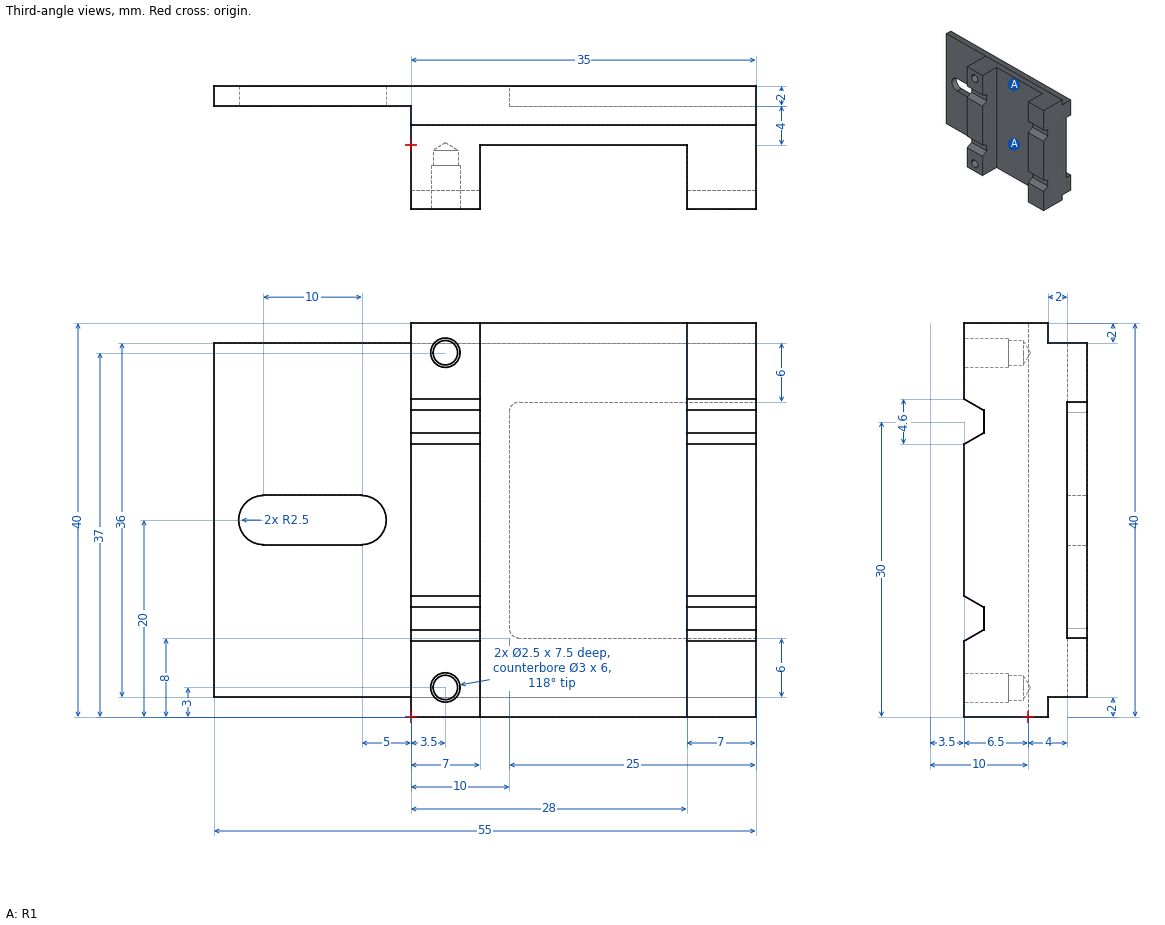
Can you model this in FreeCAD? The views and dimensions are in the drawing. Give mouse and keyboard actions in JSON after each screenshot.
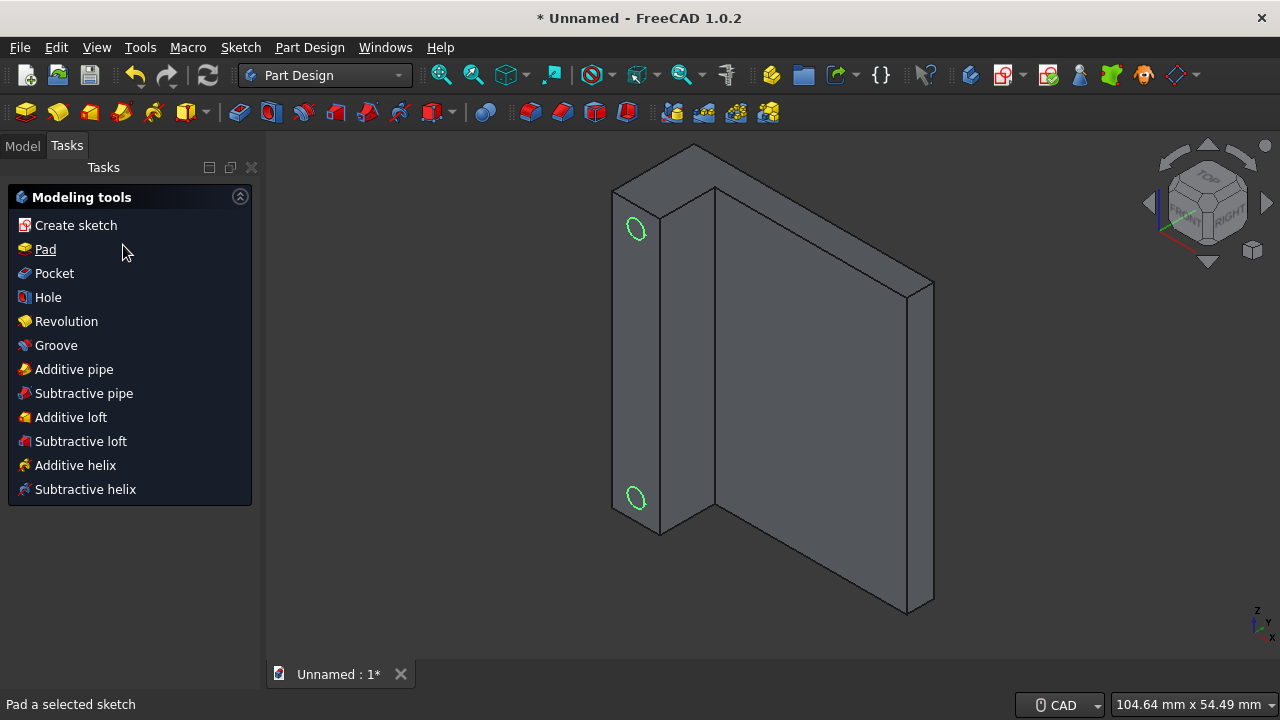
{"action": "left_click", "coordinate": [272, 112]}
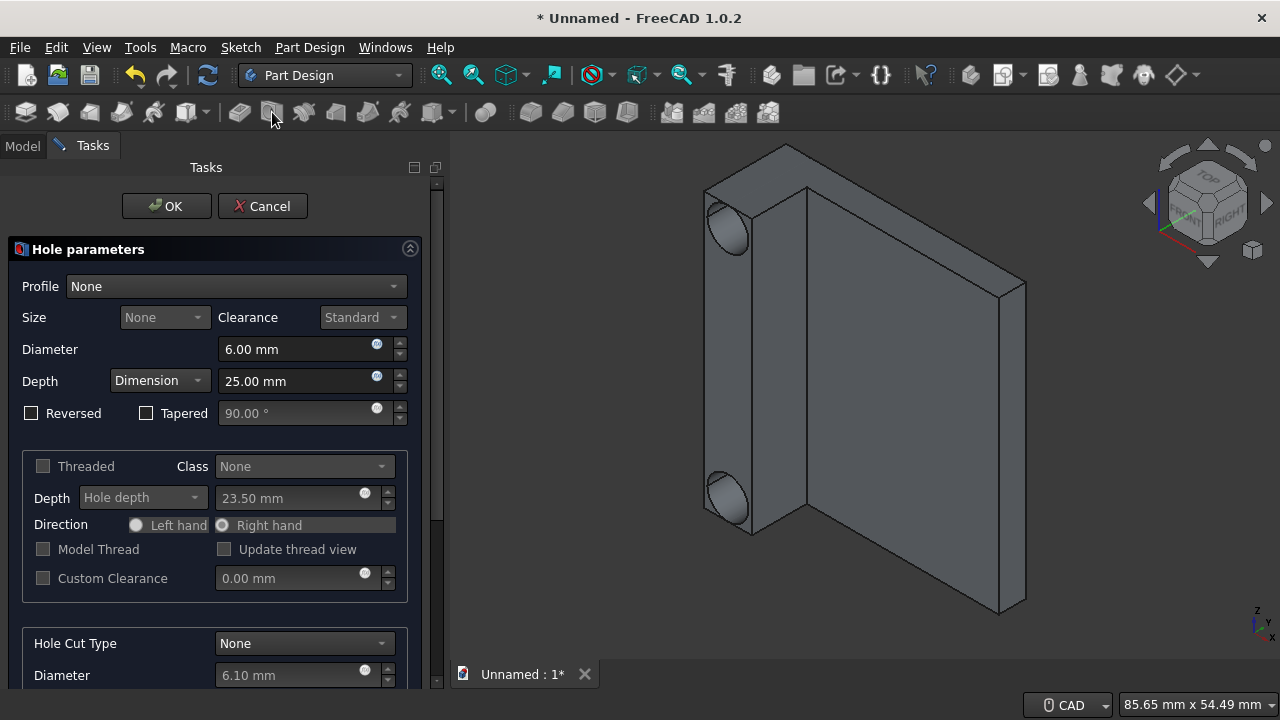
{"action": "triple_click", "coordinate": [305, 349]}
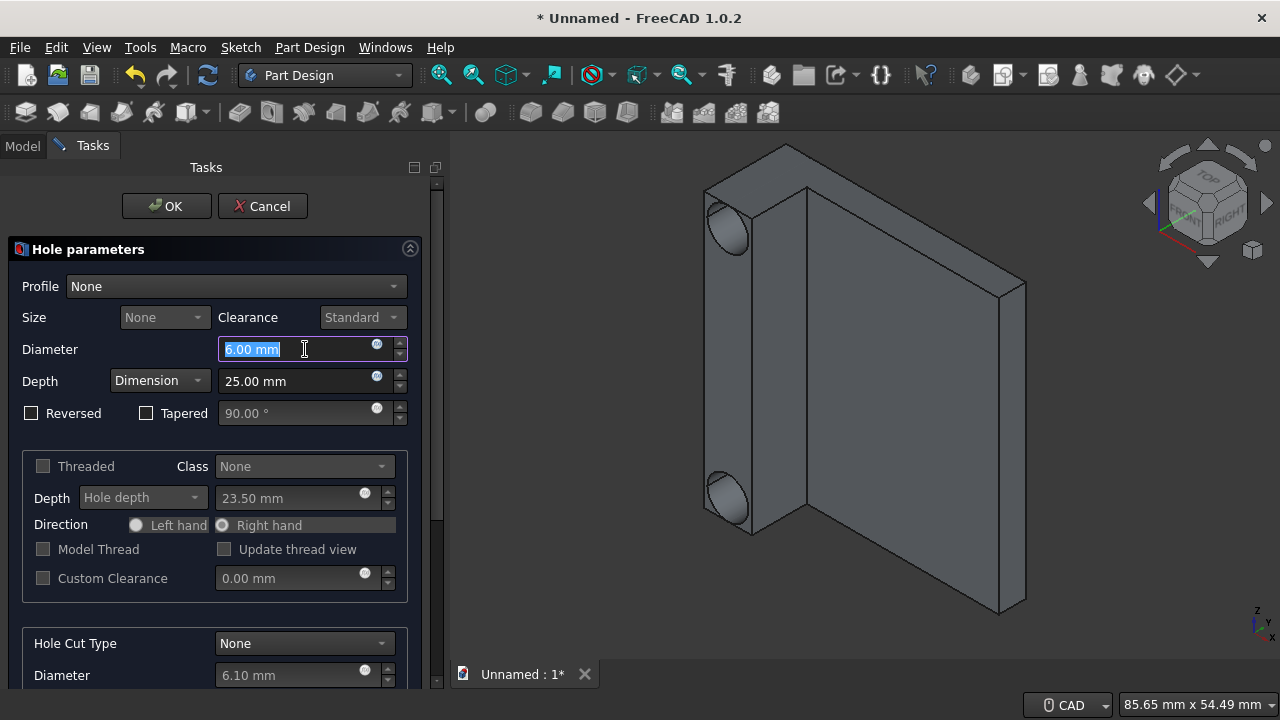
{"action": "type", "text": "2.5"}
{"action": "key", "text": "Tab"}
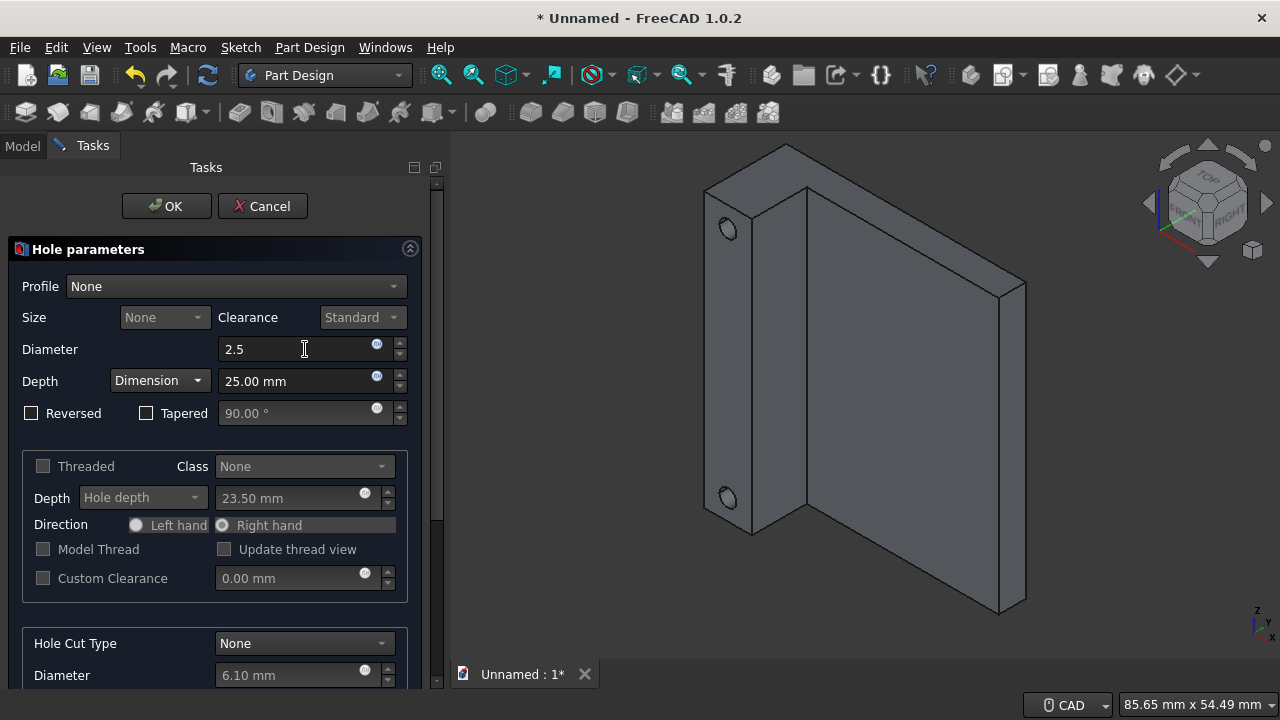
{"action": "triple_click", "coordinate": [305, 381]}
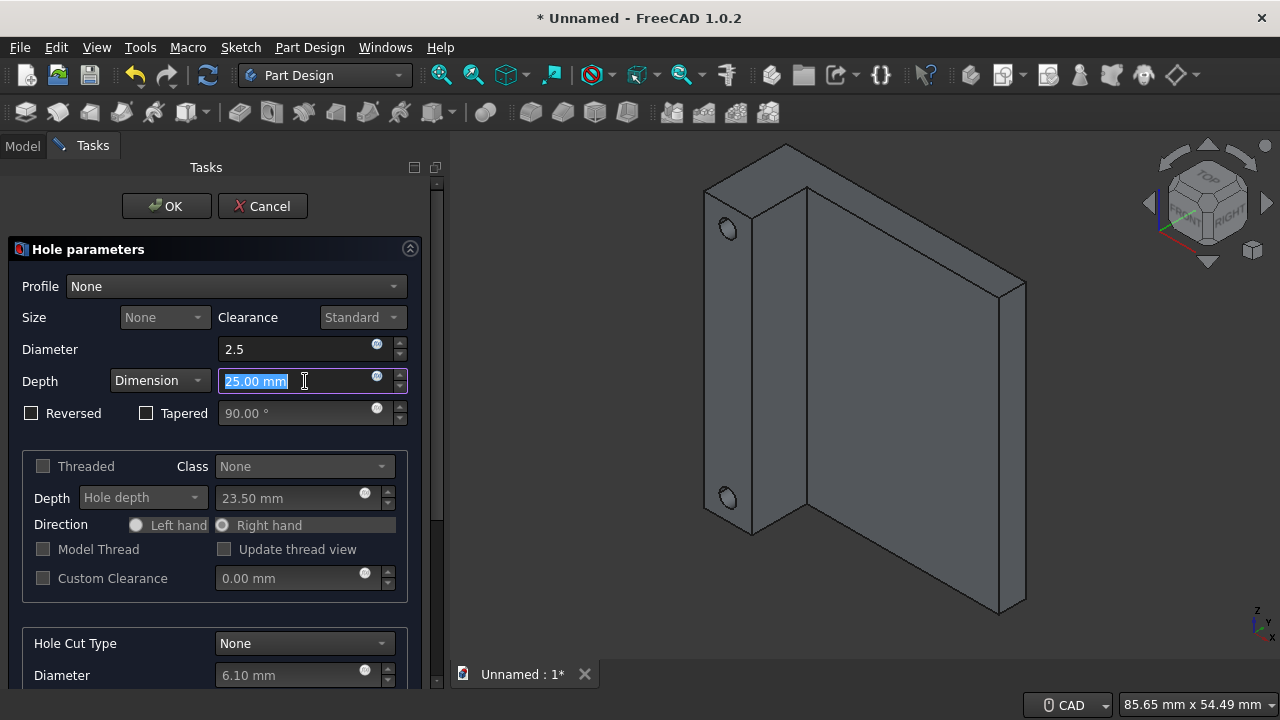
{"action": "type", "text": "7.5"}
{"action": "key", "text": "Tab"}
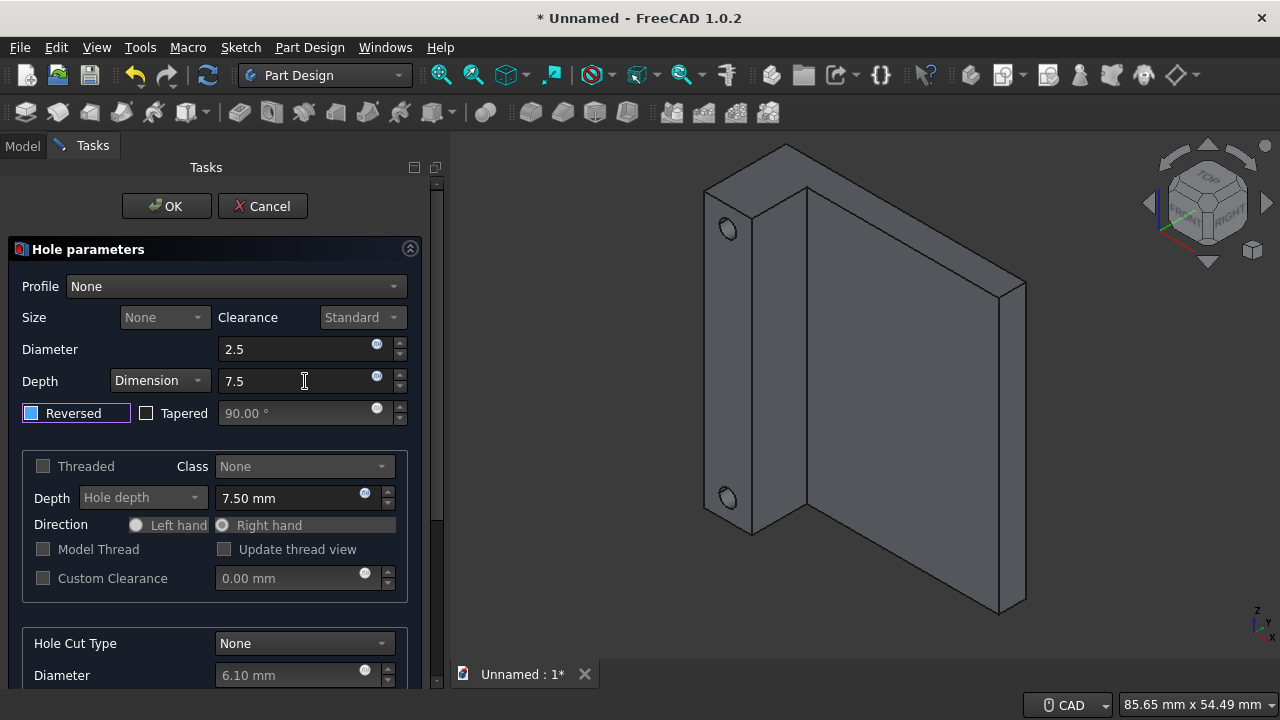
{"action": "left_click", "coordinate": [306, 644]}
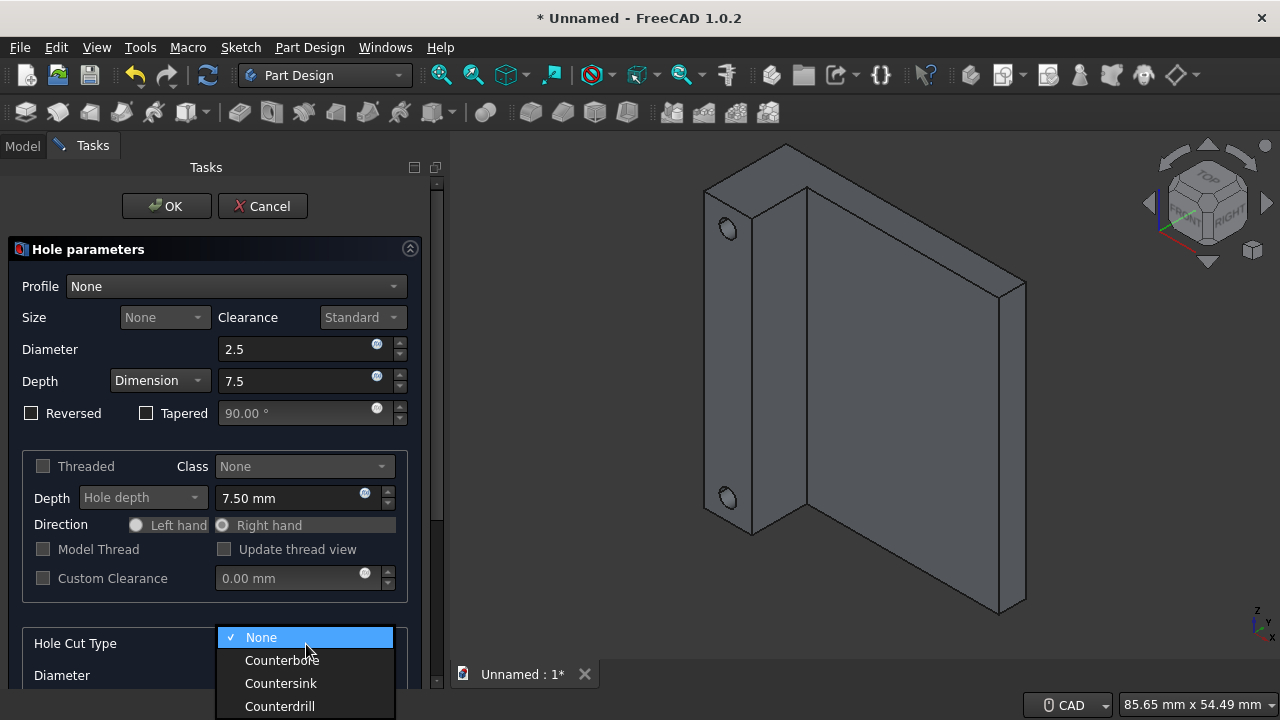
{"action": "left_click", "coordinate": [304, 660]}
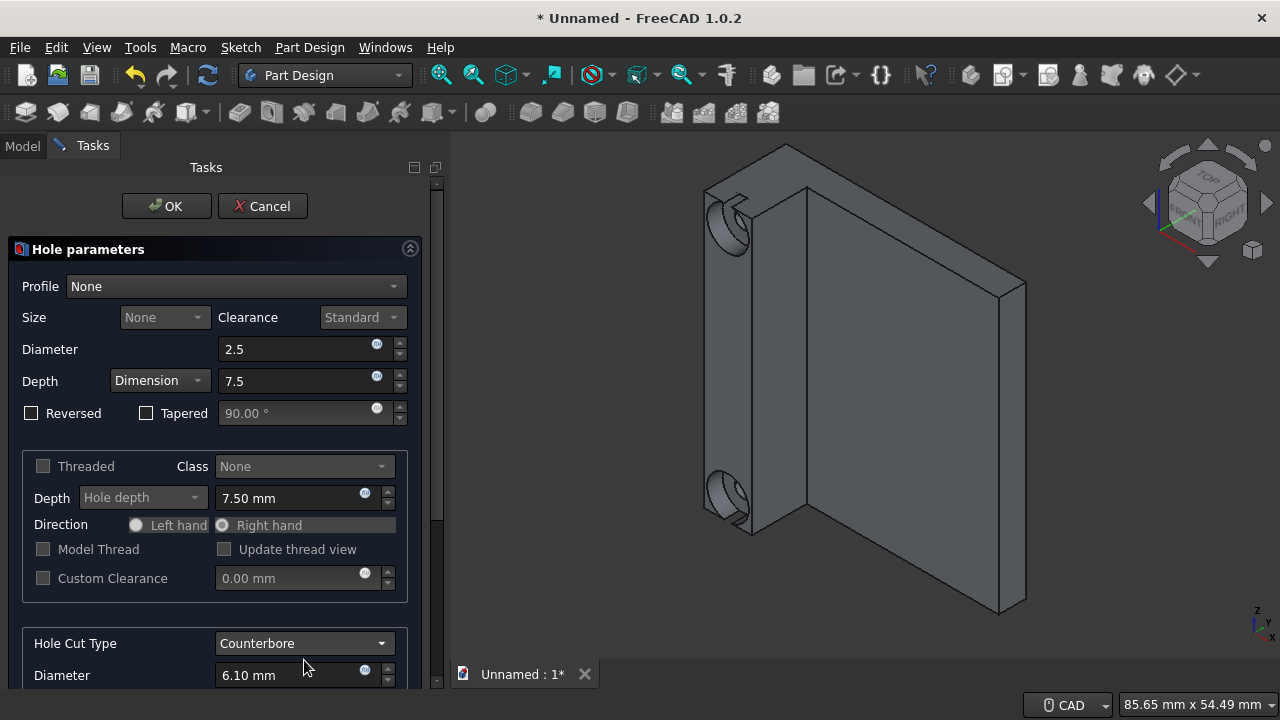
{"action": "triple_click", "coordinate": [298, 675]}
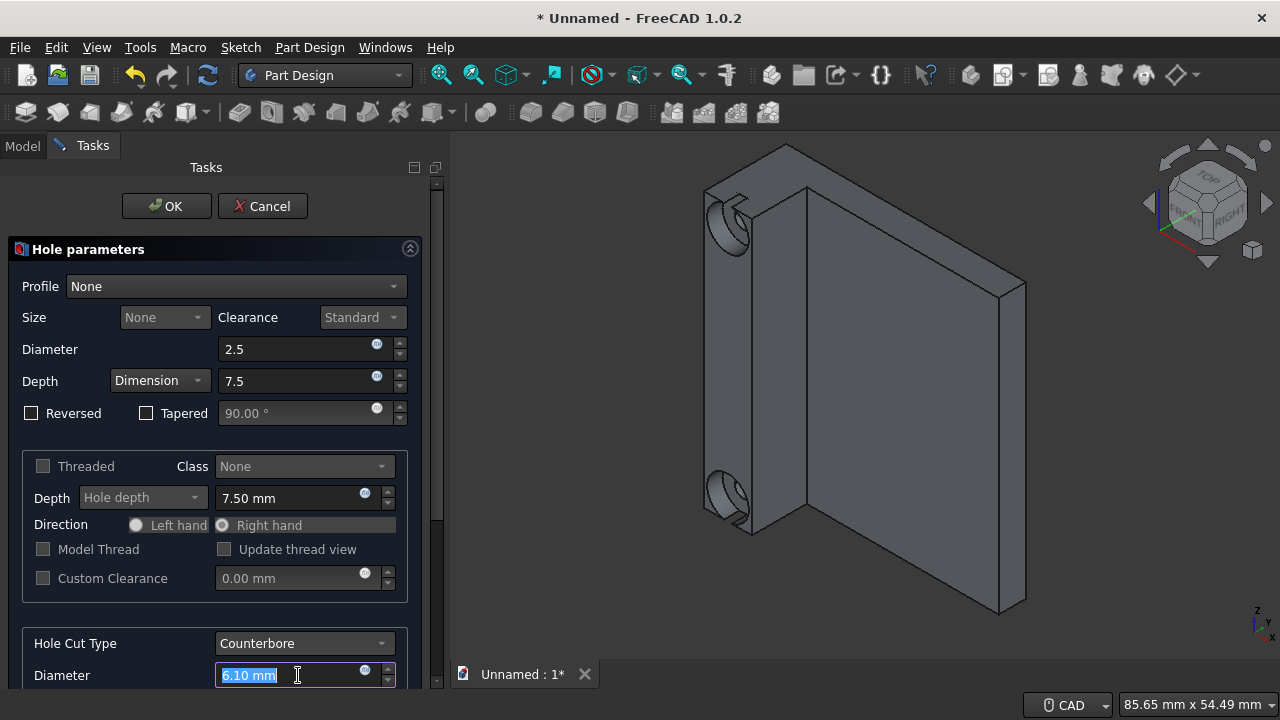
{"action": "type", "text": "3"}
{"action": "key", "text": "Tab"}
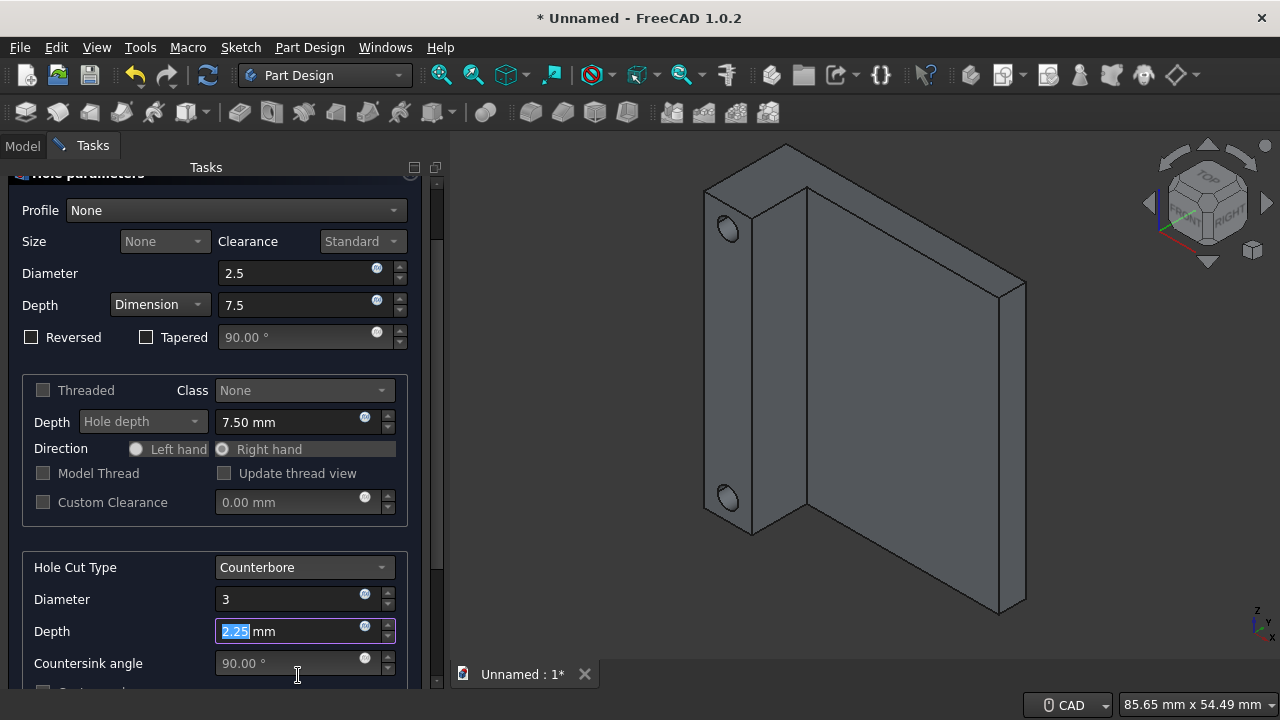
{"action": "type", "text": "6"}
{"action": "key", "text": "Tab"}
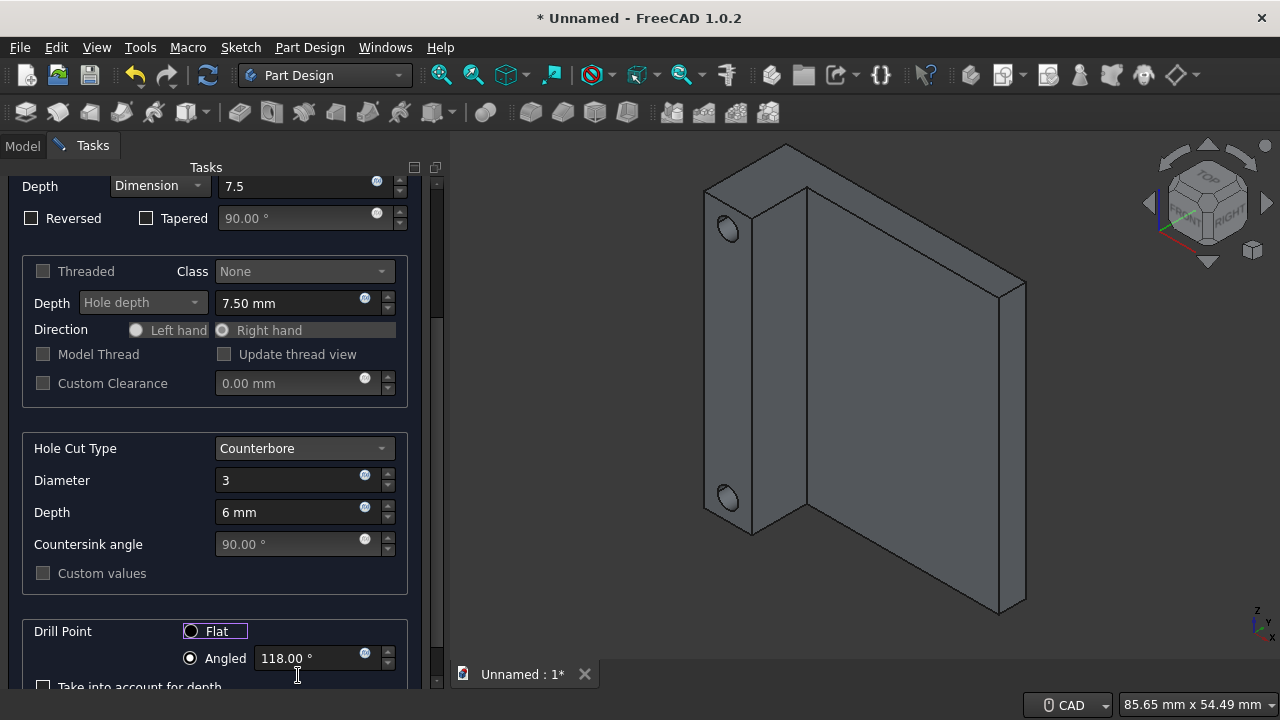
{"action": "scroll", "coordinate": [437, 432], "scroll_direction": "up", "scroll_amount": 4}